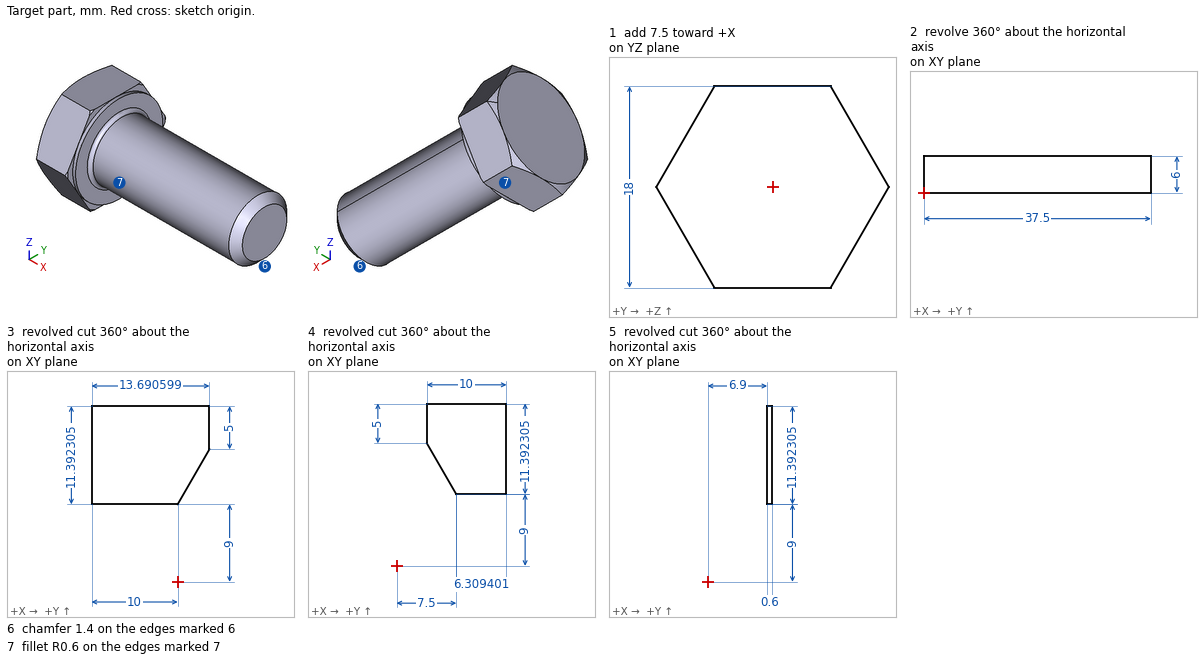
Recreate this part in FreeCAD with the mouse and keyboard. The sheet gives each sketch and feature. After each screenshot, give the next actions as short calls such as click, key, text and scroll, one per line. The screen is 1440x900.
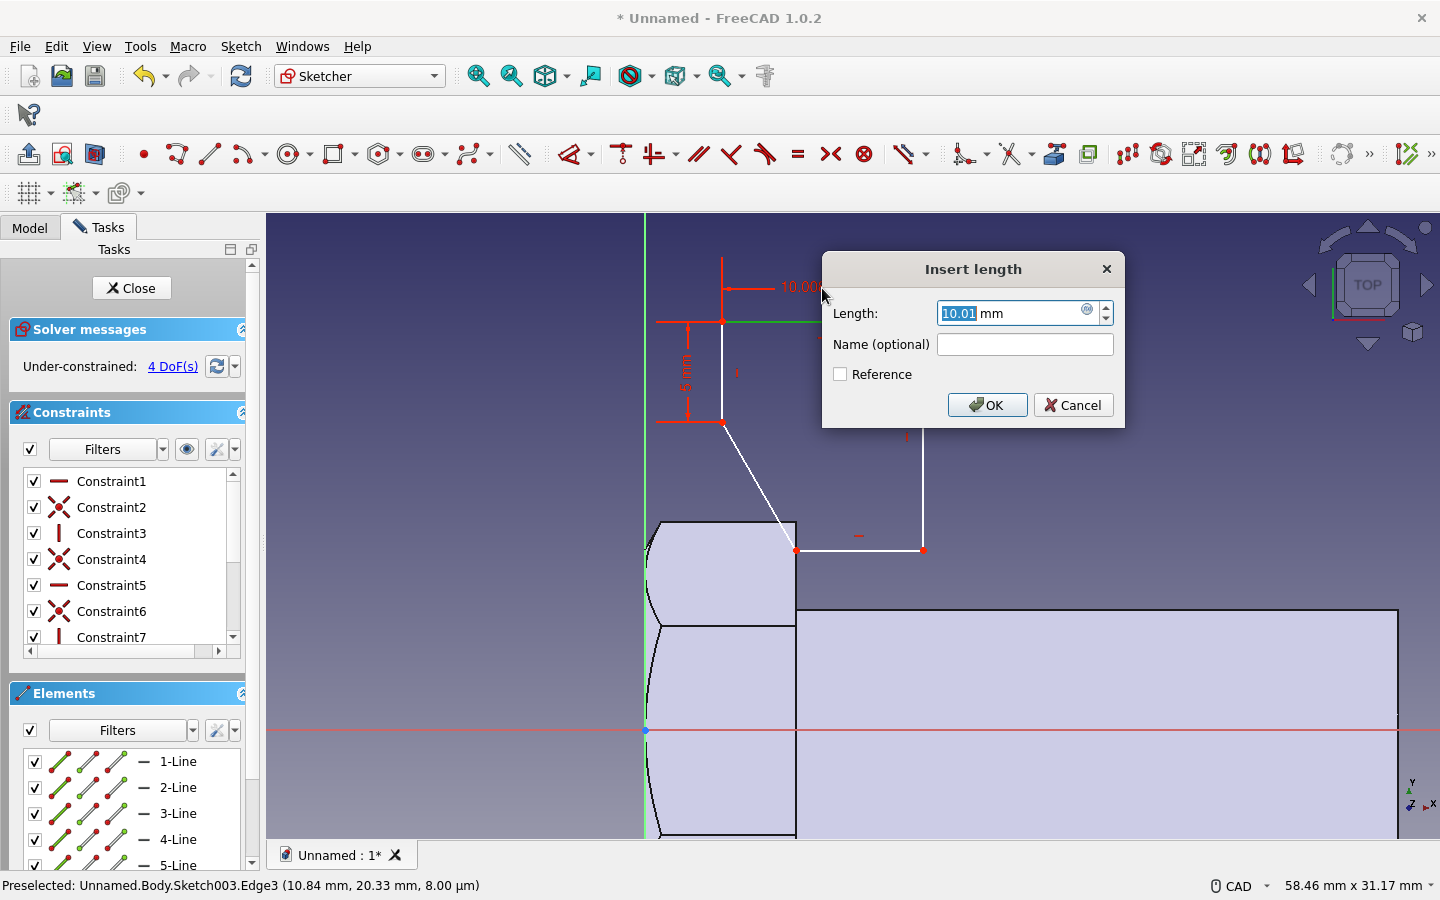
text(10)
key(Return)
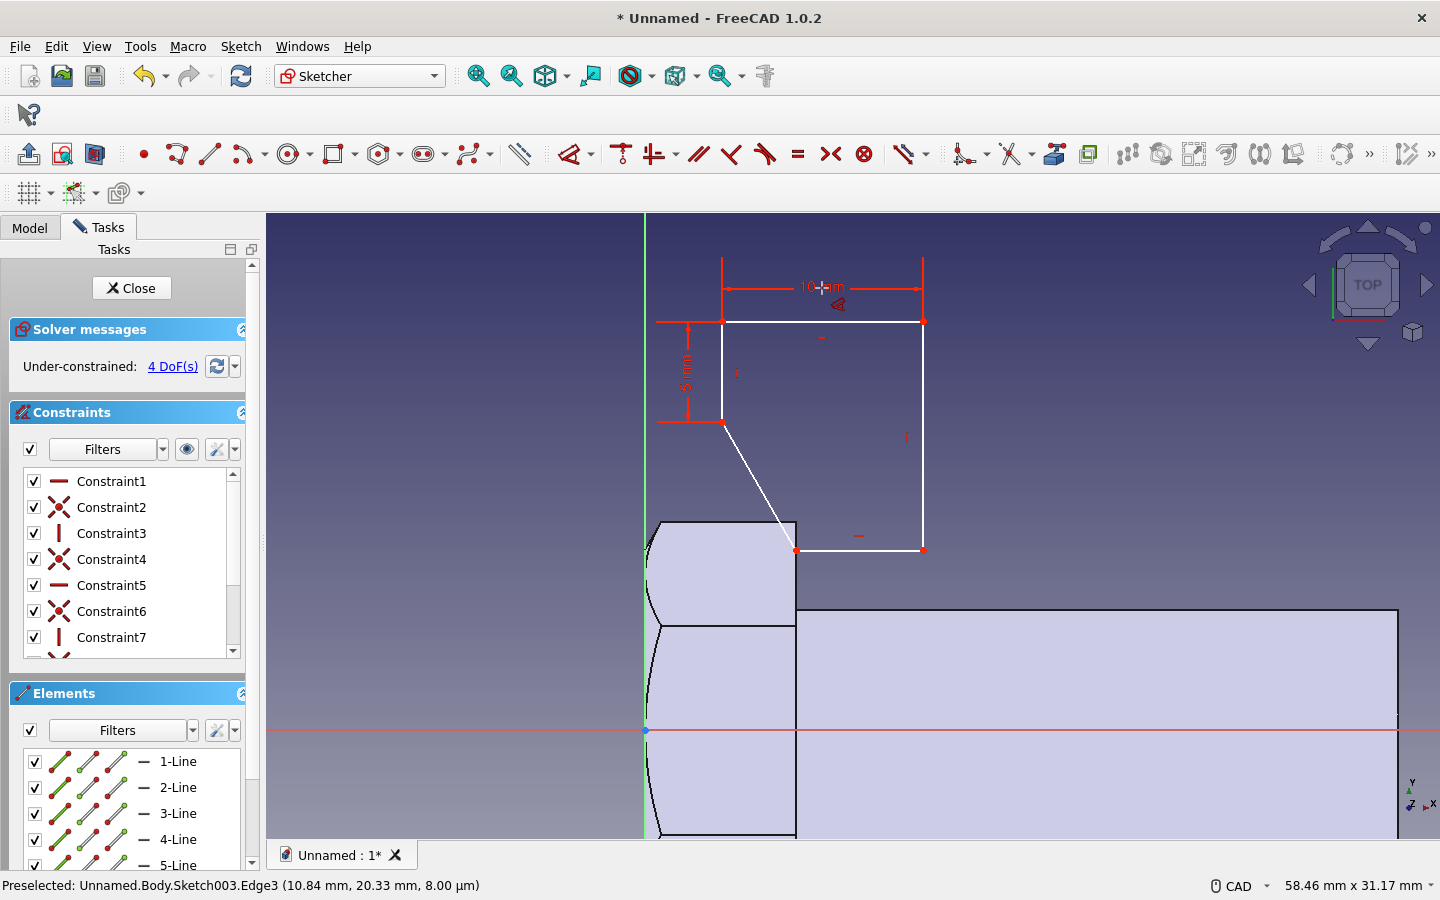
click(796, 551)
click(611, 641)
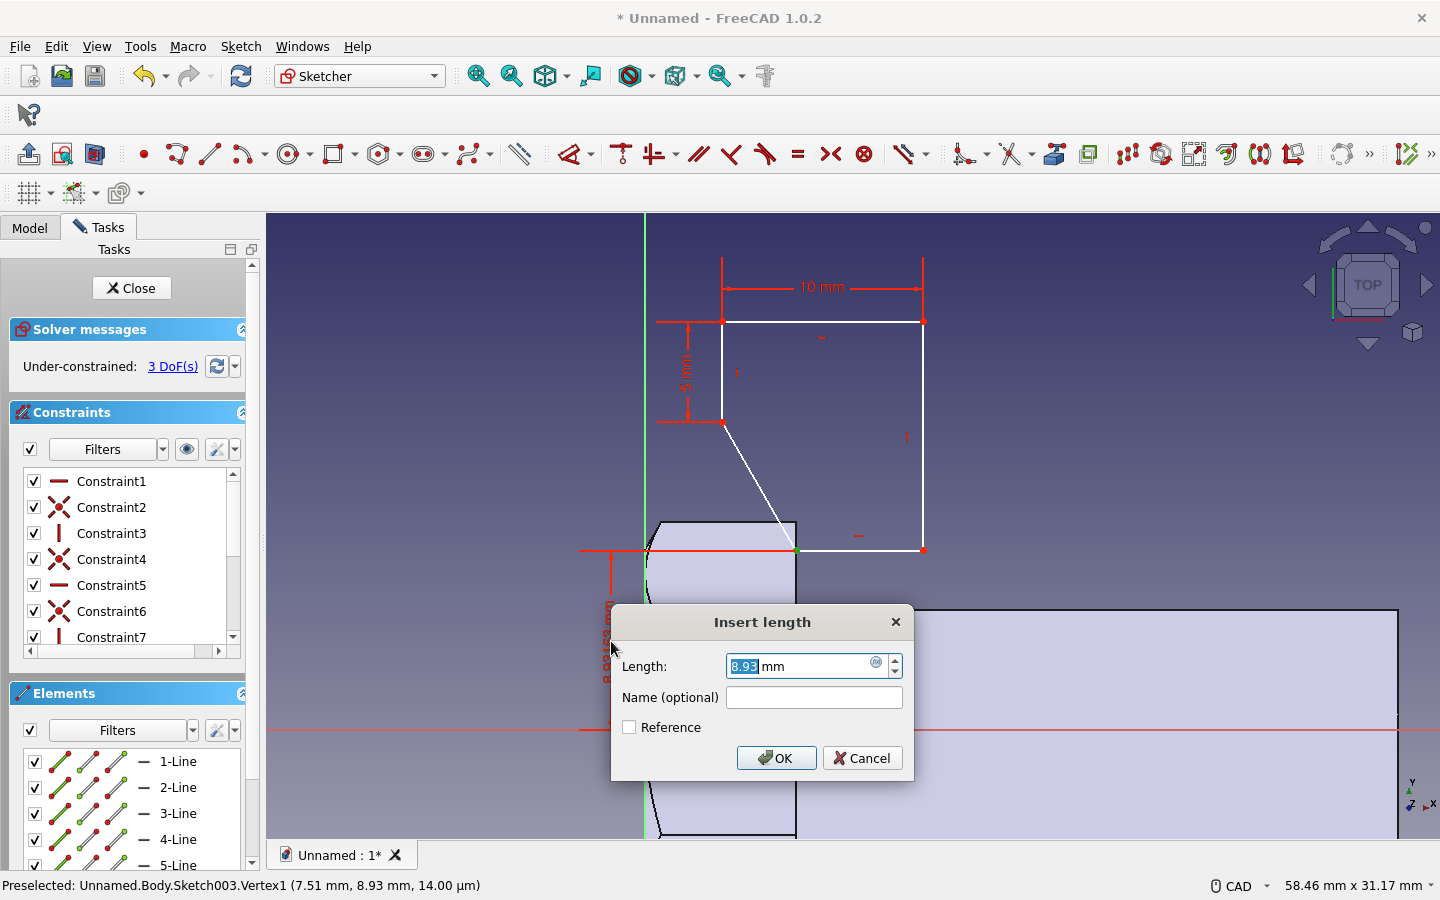
text(9)
key(Return)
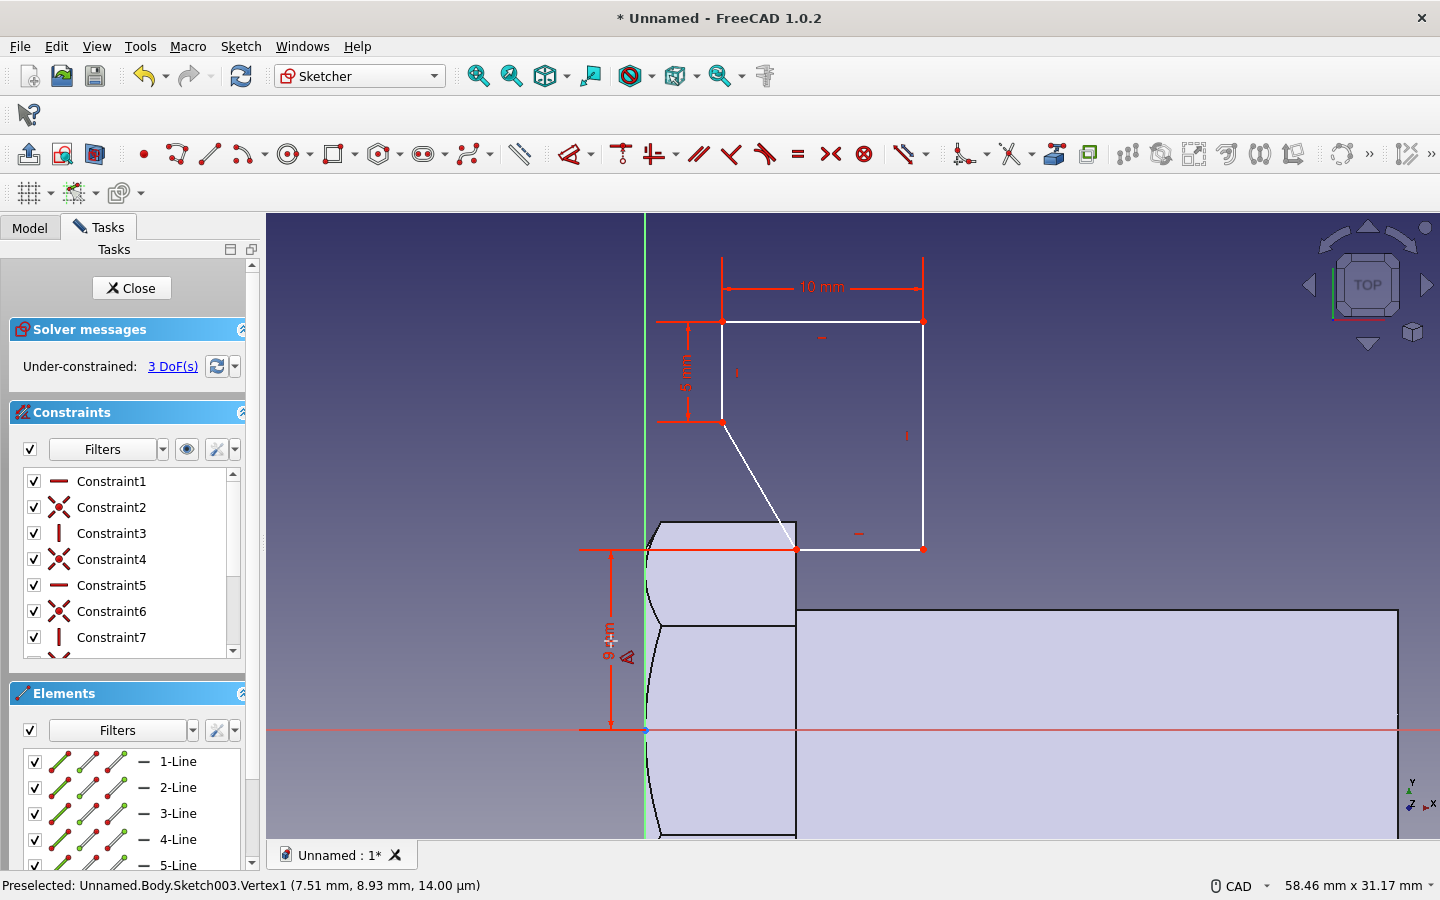
click(796, 550)
click(721, 764)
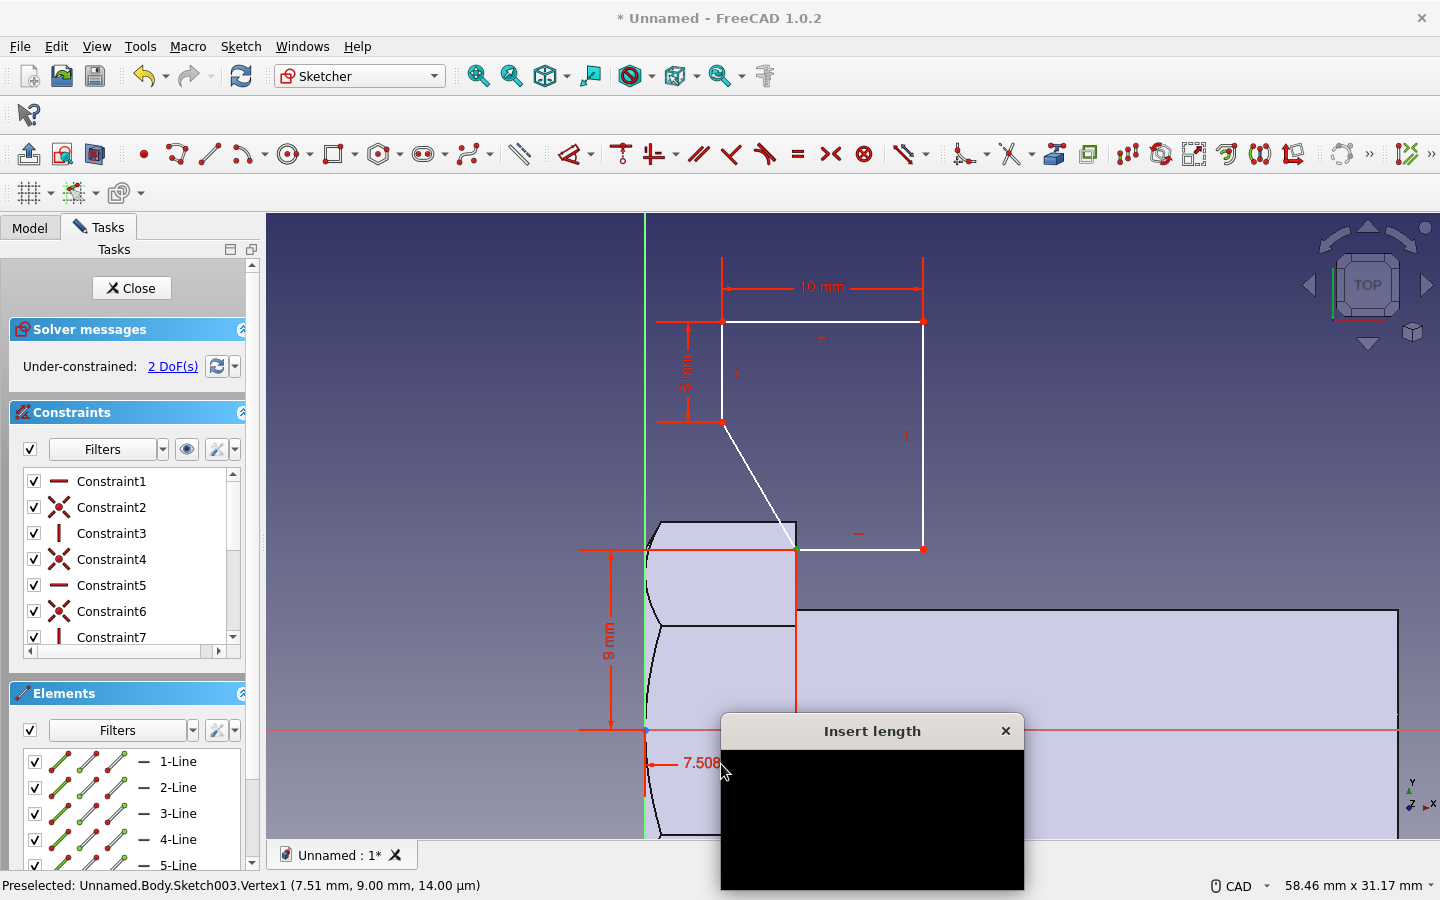
text(7.5)
key(Return)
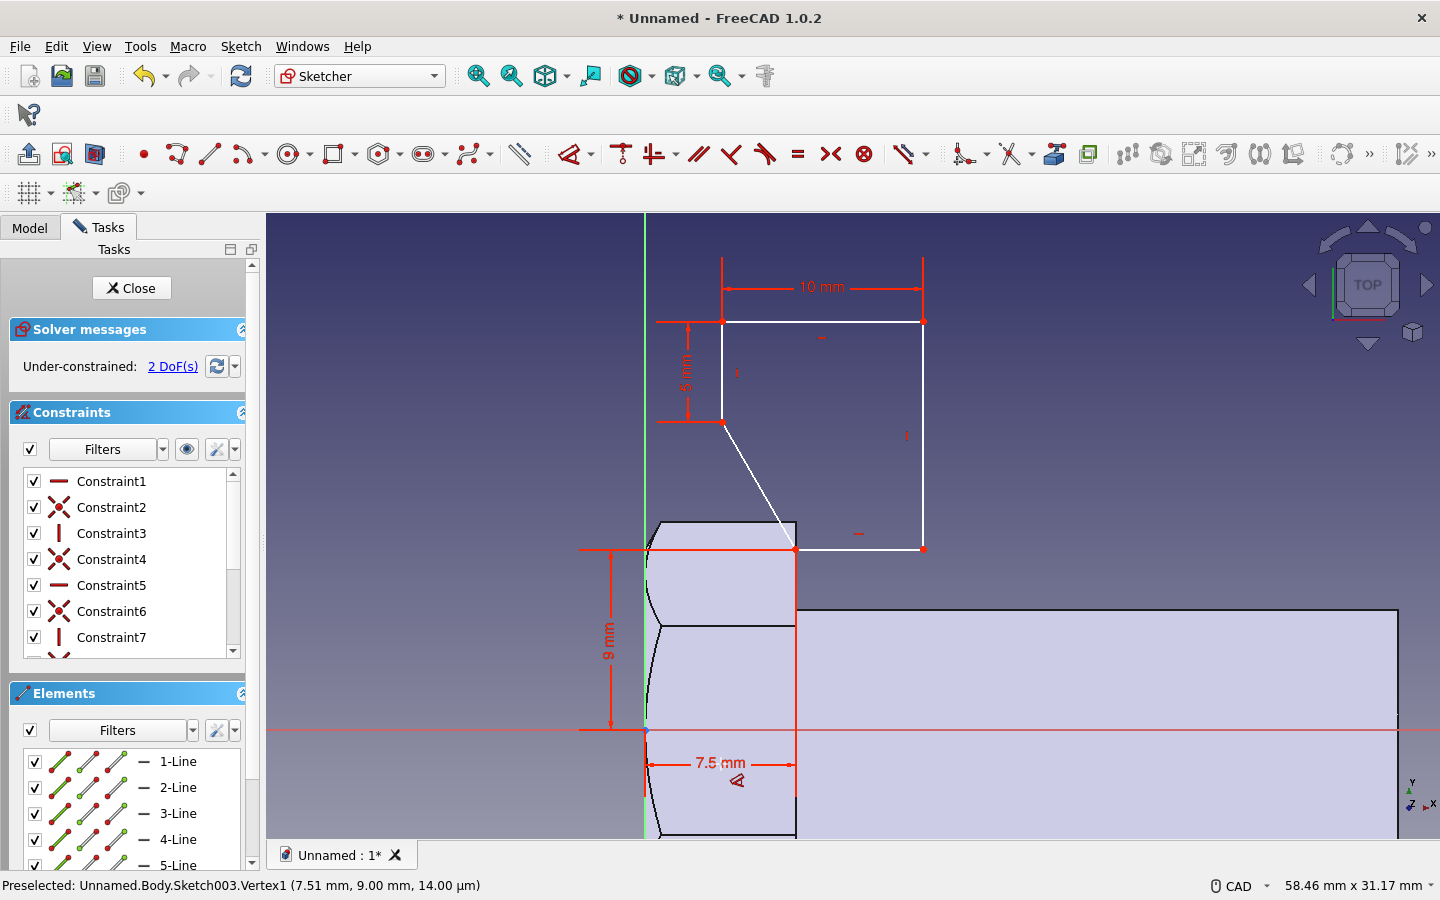
click(834, 550)
click(859, 584)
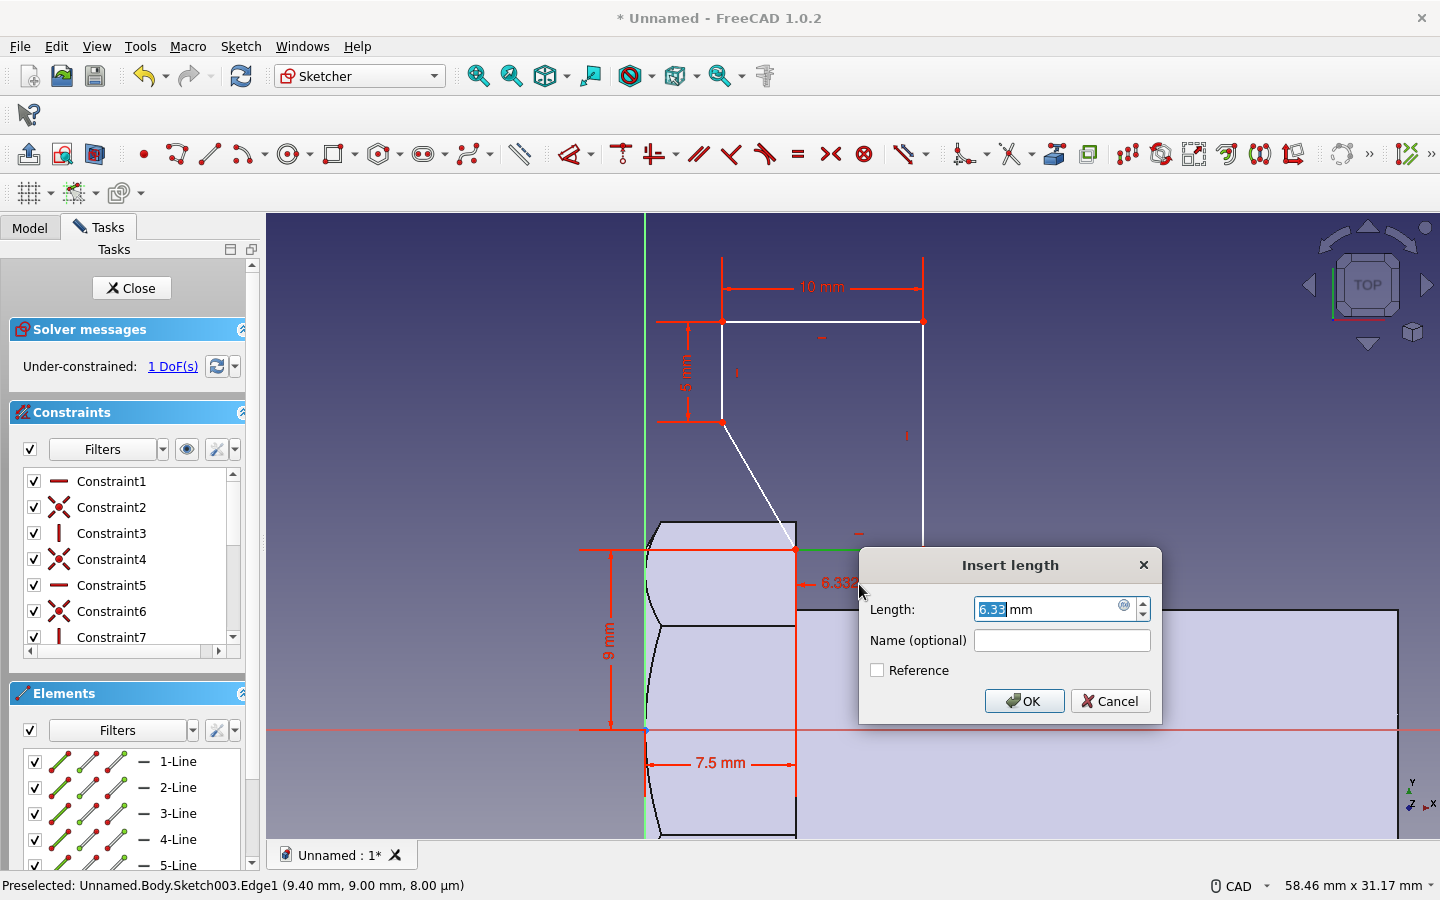
text(6.309401)
key(Return)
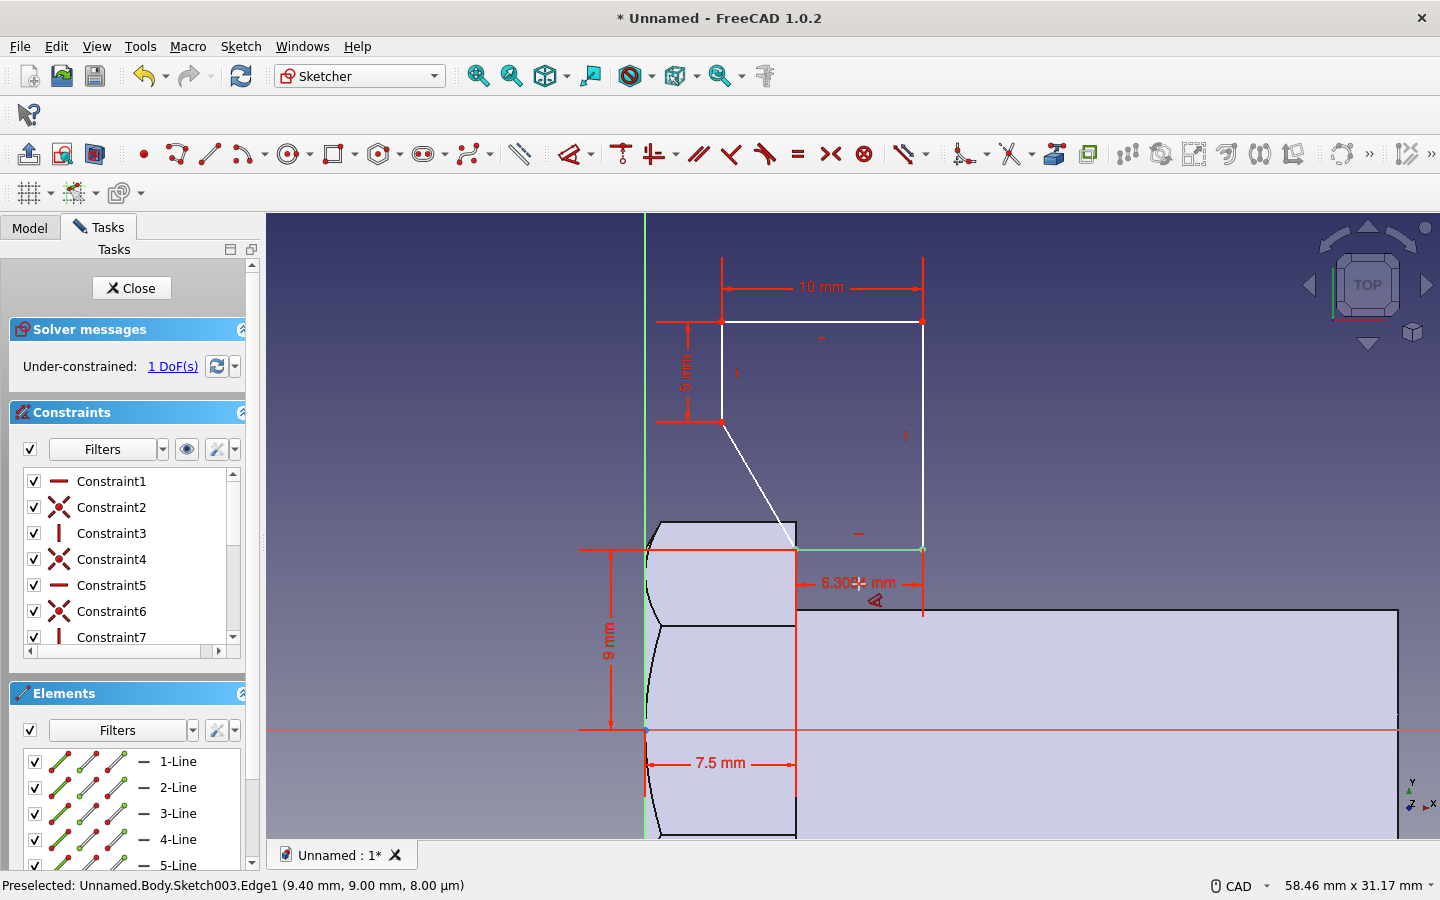
click(923, 481)
click(957, 436)